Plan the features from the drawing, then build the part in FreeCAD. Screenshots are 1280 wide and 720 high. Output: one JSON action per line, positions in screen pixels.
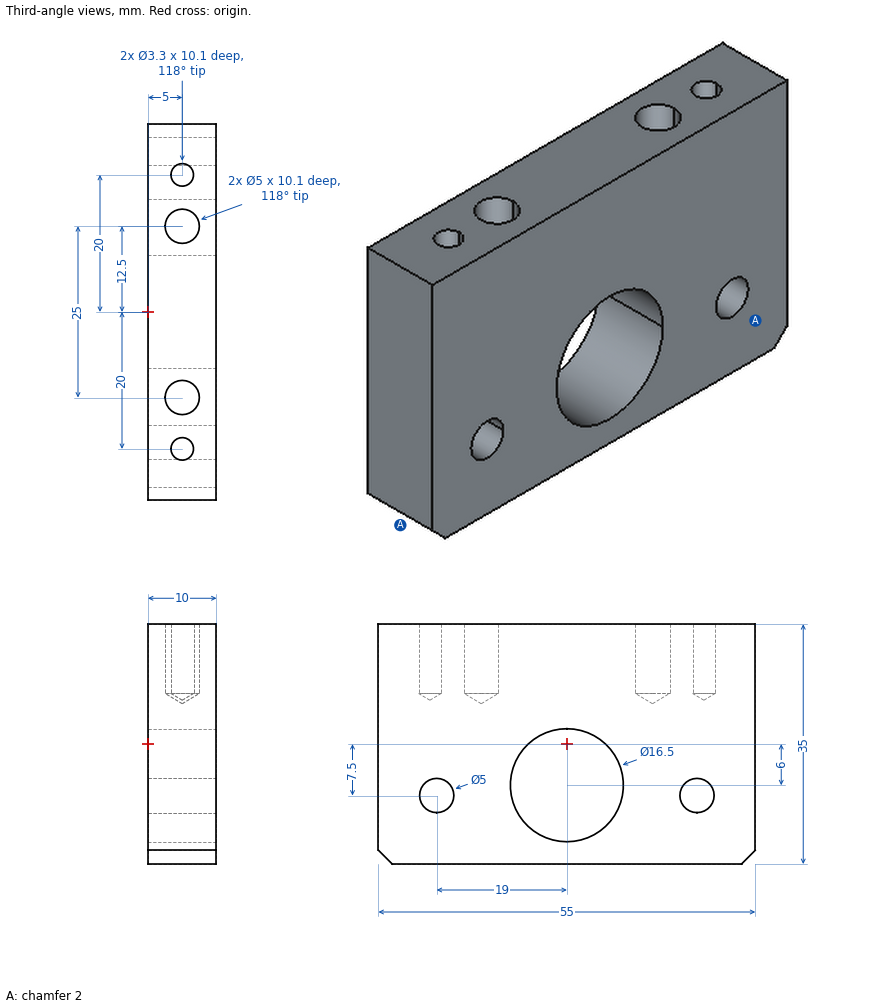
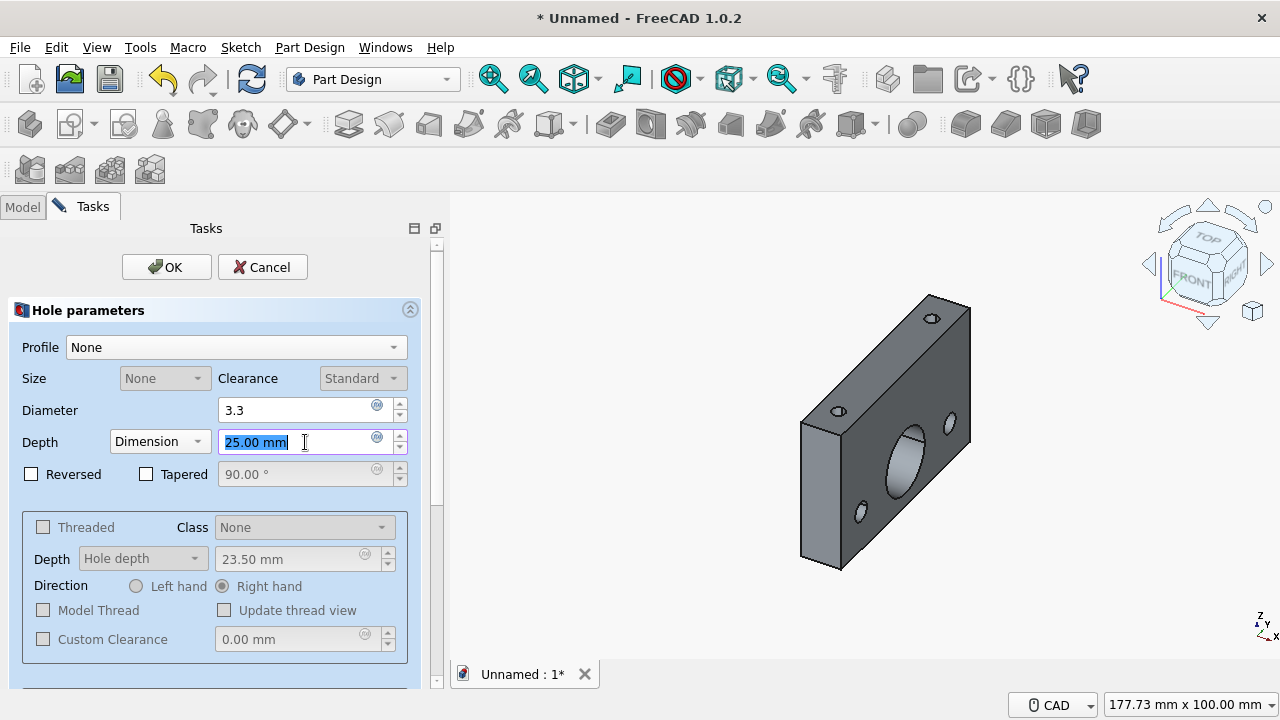
{"action": "type", "text": "10.1"}
{"action": "key", "text": "Tab"}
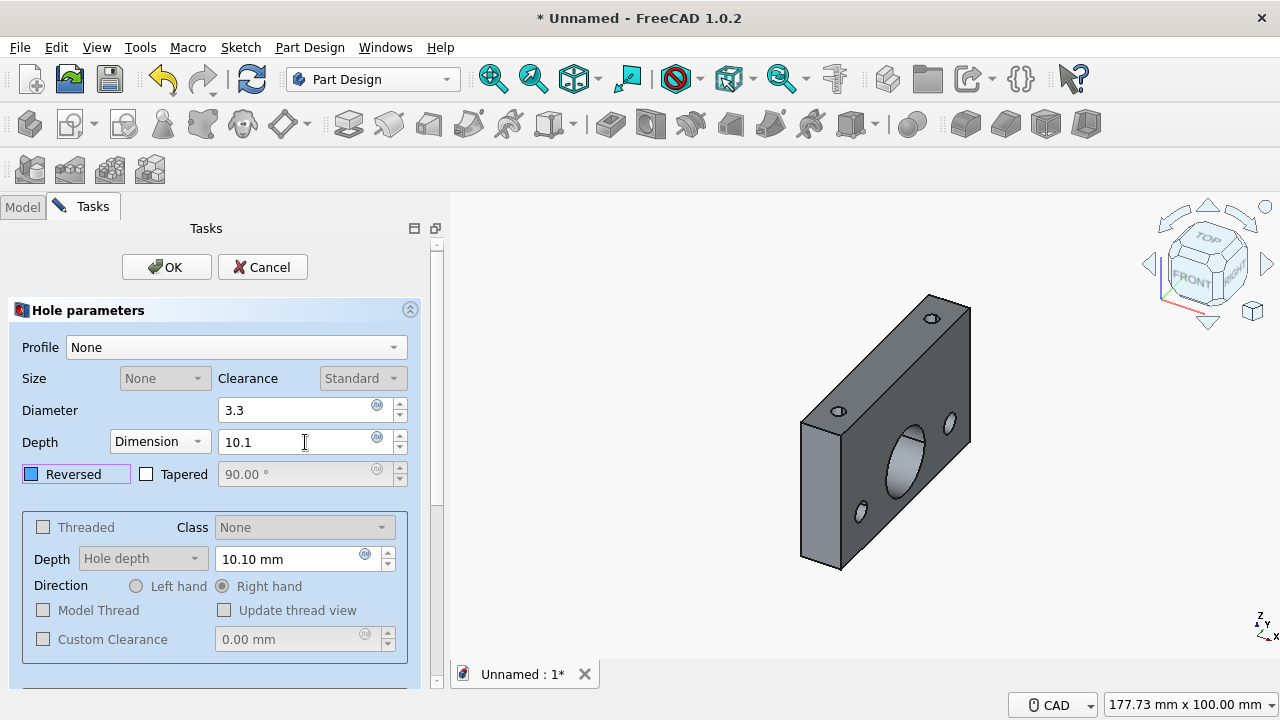
{"action": "left_click", "coordinate": [167, 267]}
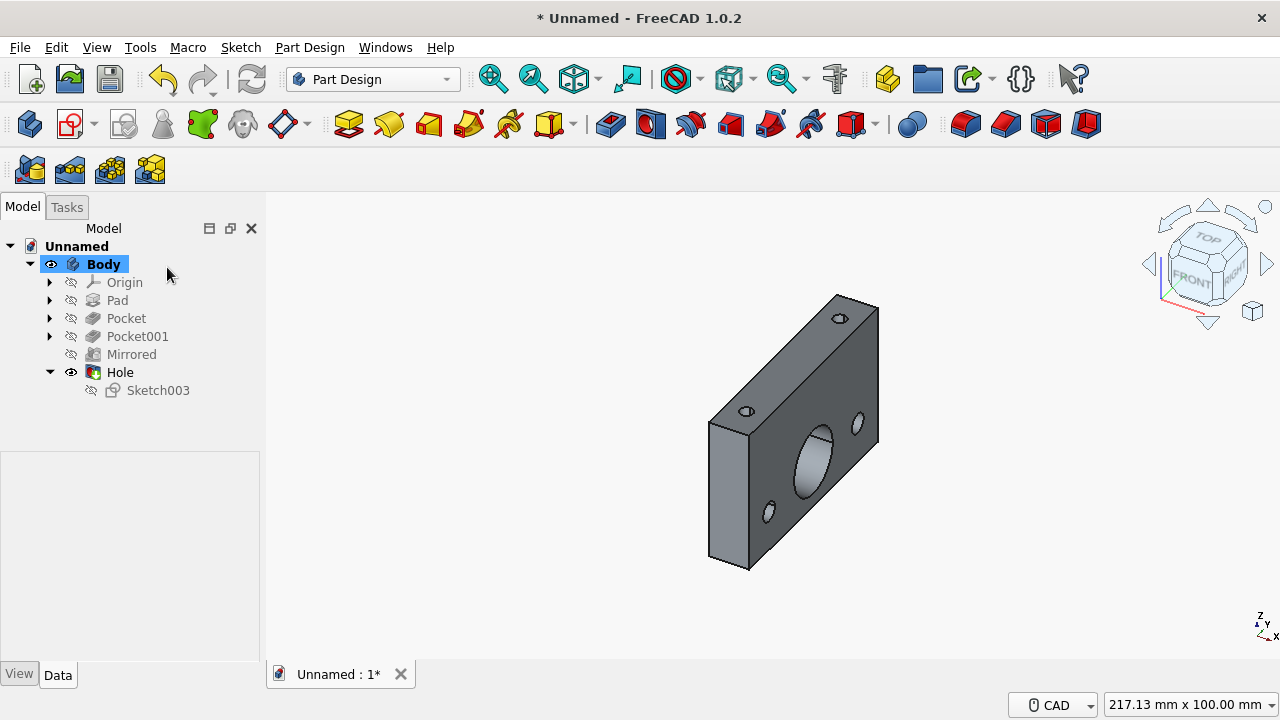
{"action": "left_click", "coordinate": [812, 346]}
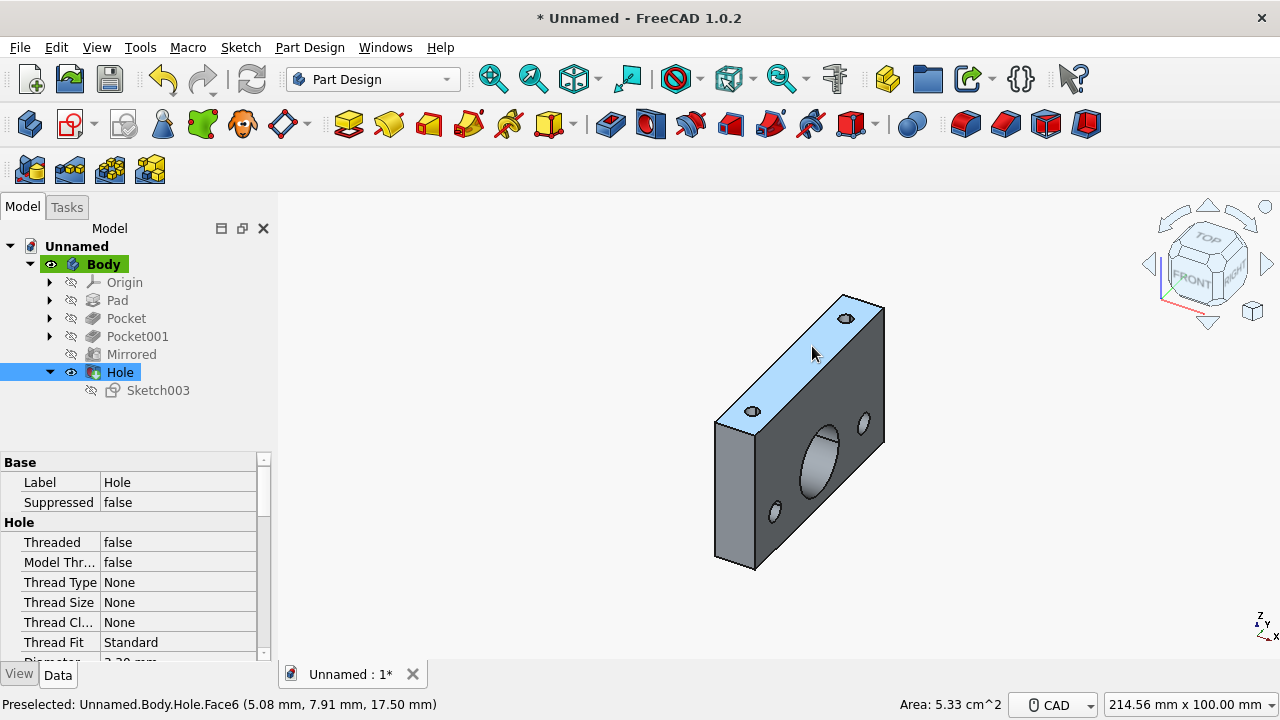
{"action": "left_click", "coordinate": [70, 124]}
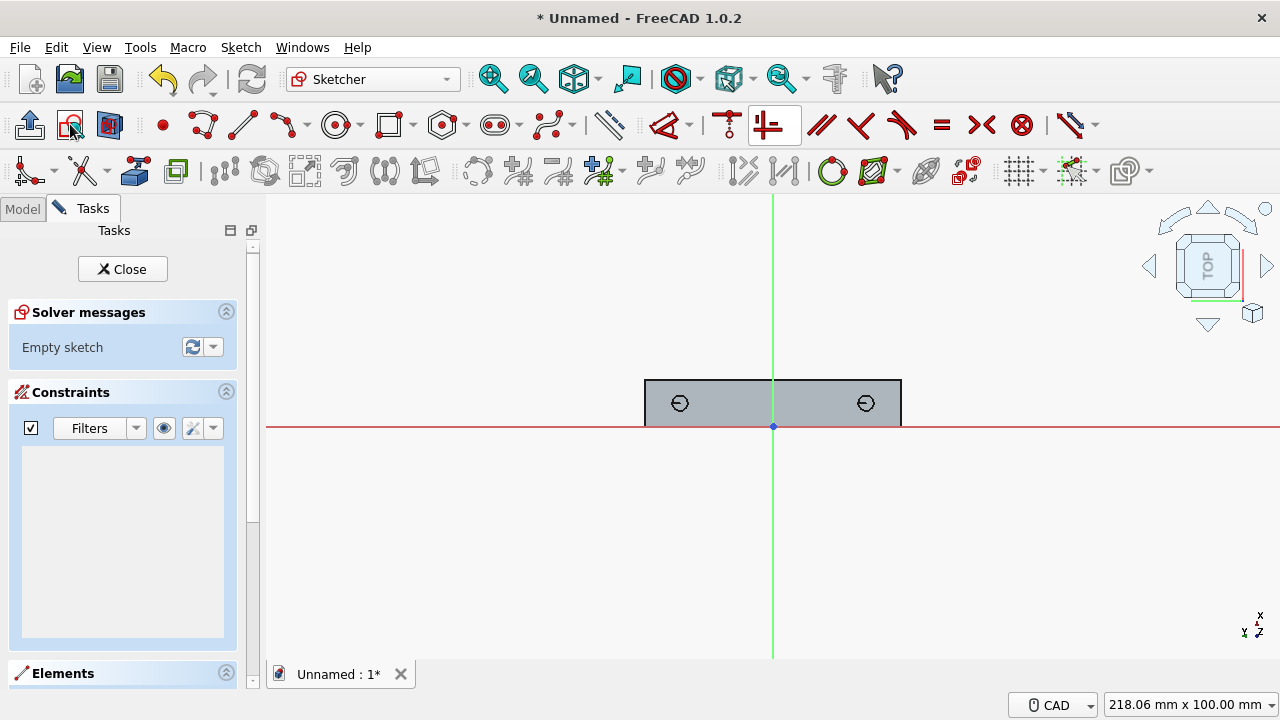
{"action": "scroll", "coordinate": [795, 403], "scroll_direction": "up", "scroll_amount": 7}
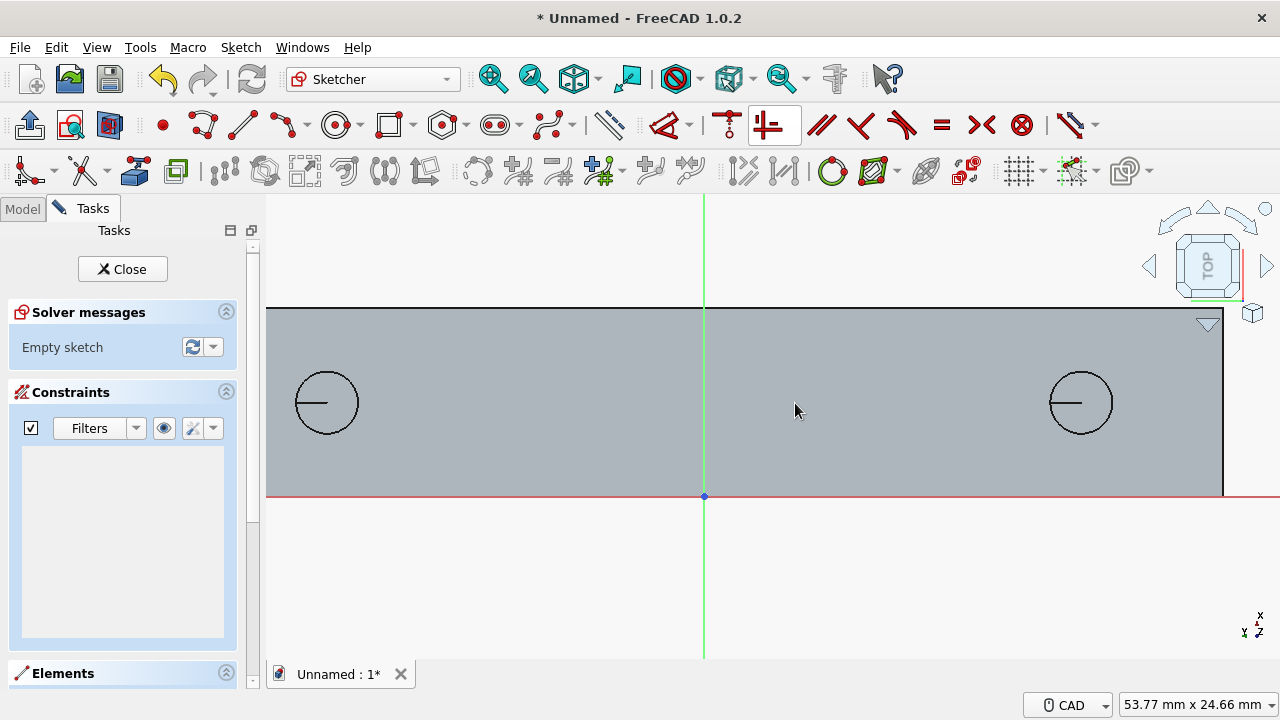
{"action": "key", "text": "g c"}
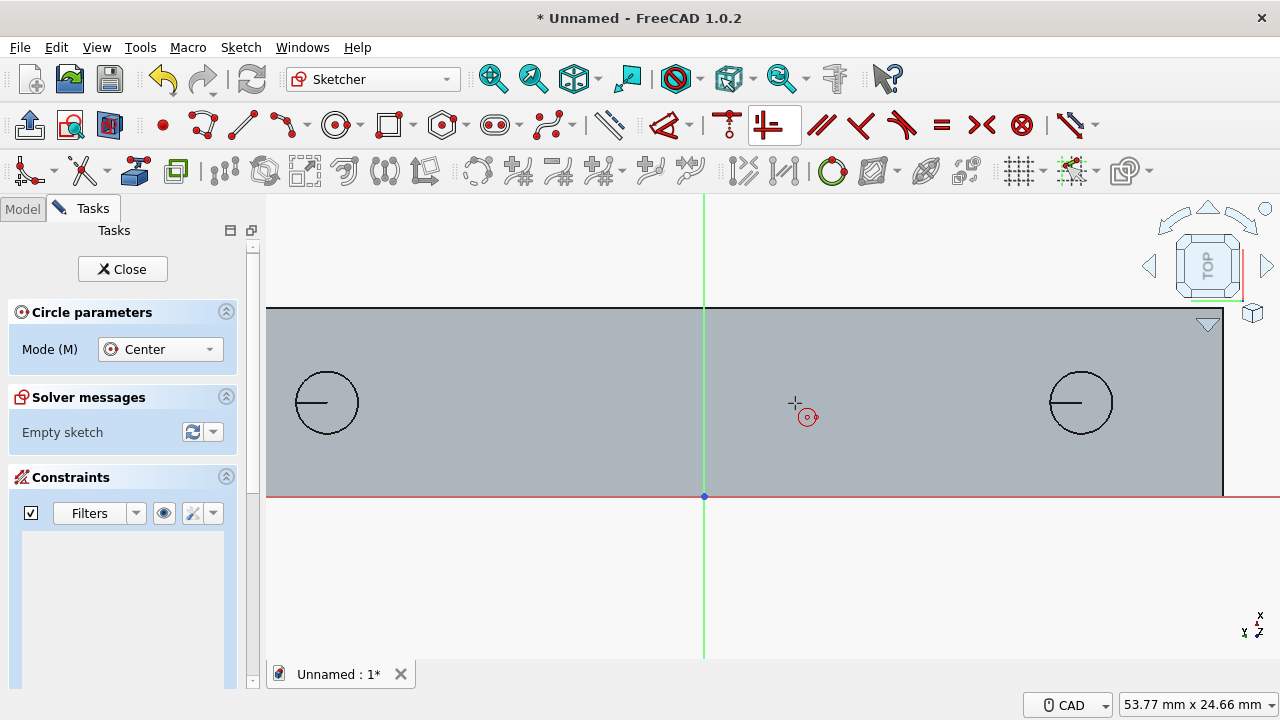
{"action": "left_click", "coordinate": [468, 403]}
{"action": "mouse_move", "coordinate": [502, 369]}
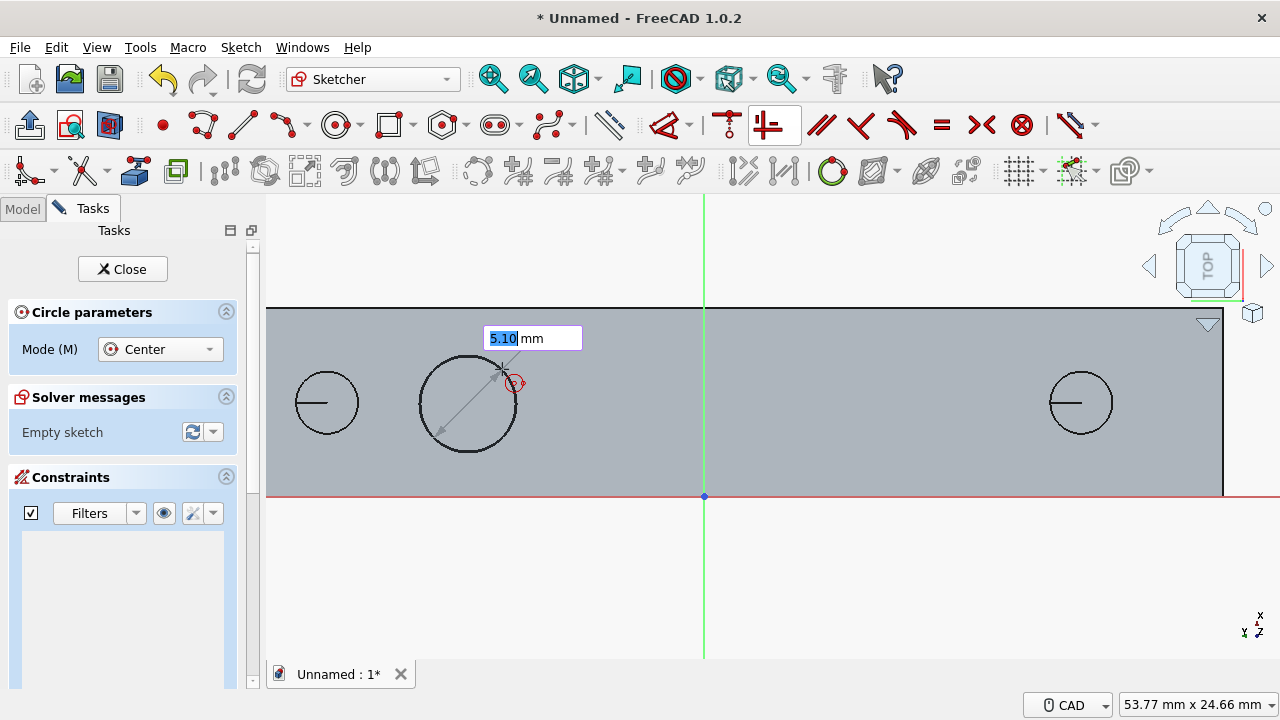
{"action": "type", "text": "5"}
{"action": "key", "text": "Return"}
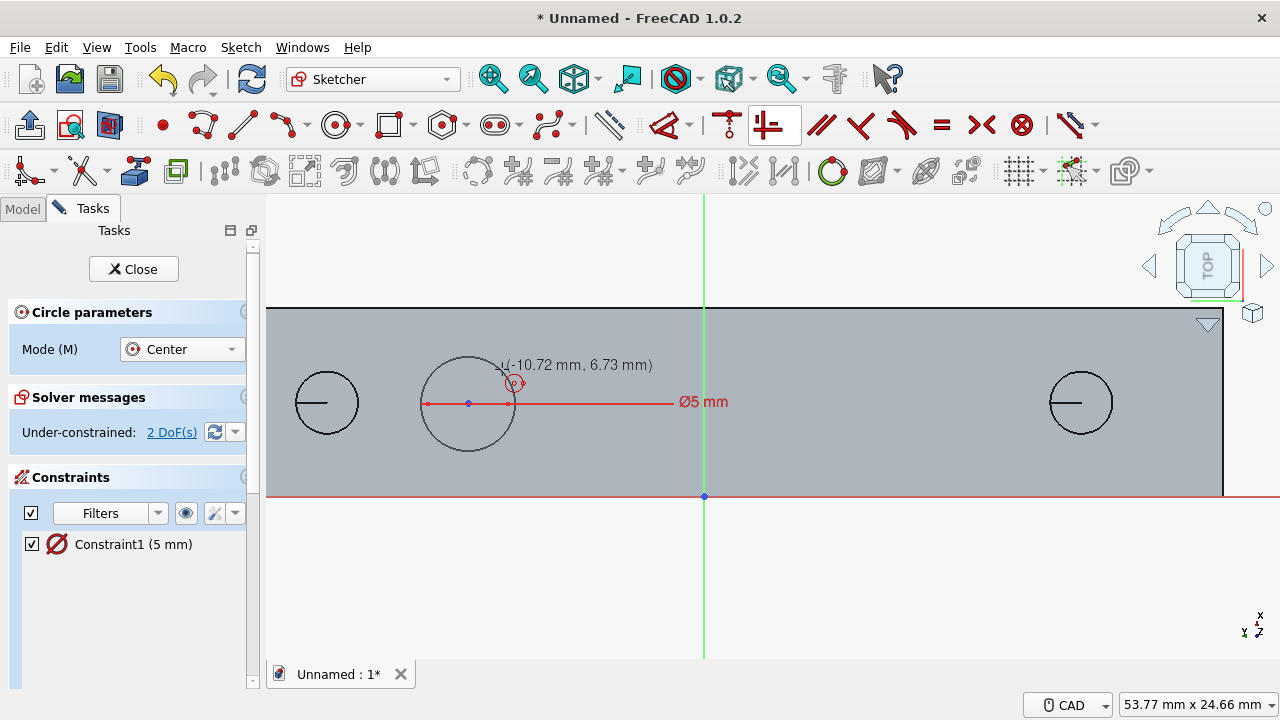
{"action": "left_click", "coordinate": [940, 403]}
{"action": "mouse_move", "coordinate": [973, 369]}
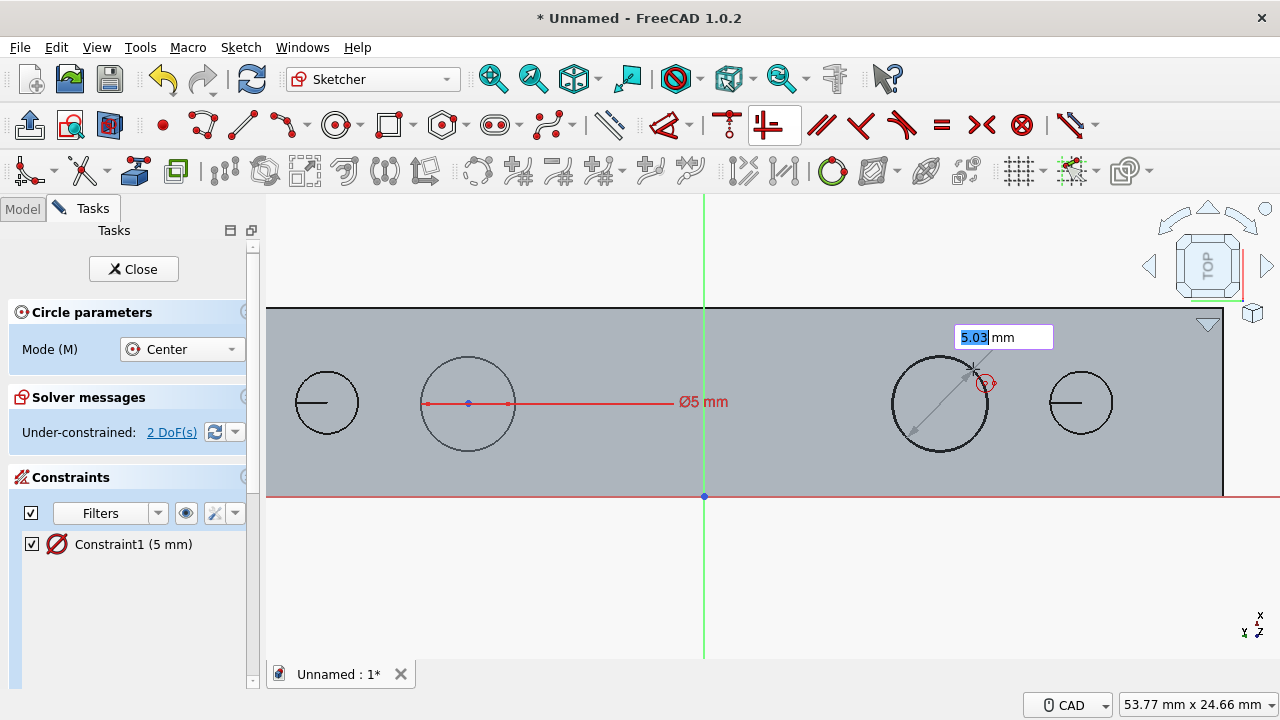
{"action": "type", "text": "5"}
{"action": "key", "text": "Return"}
{"action": "key", "text": "Escape"}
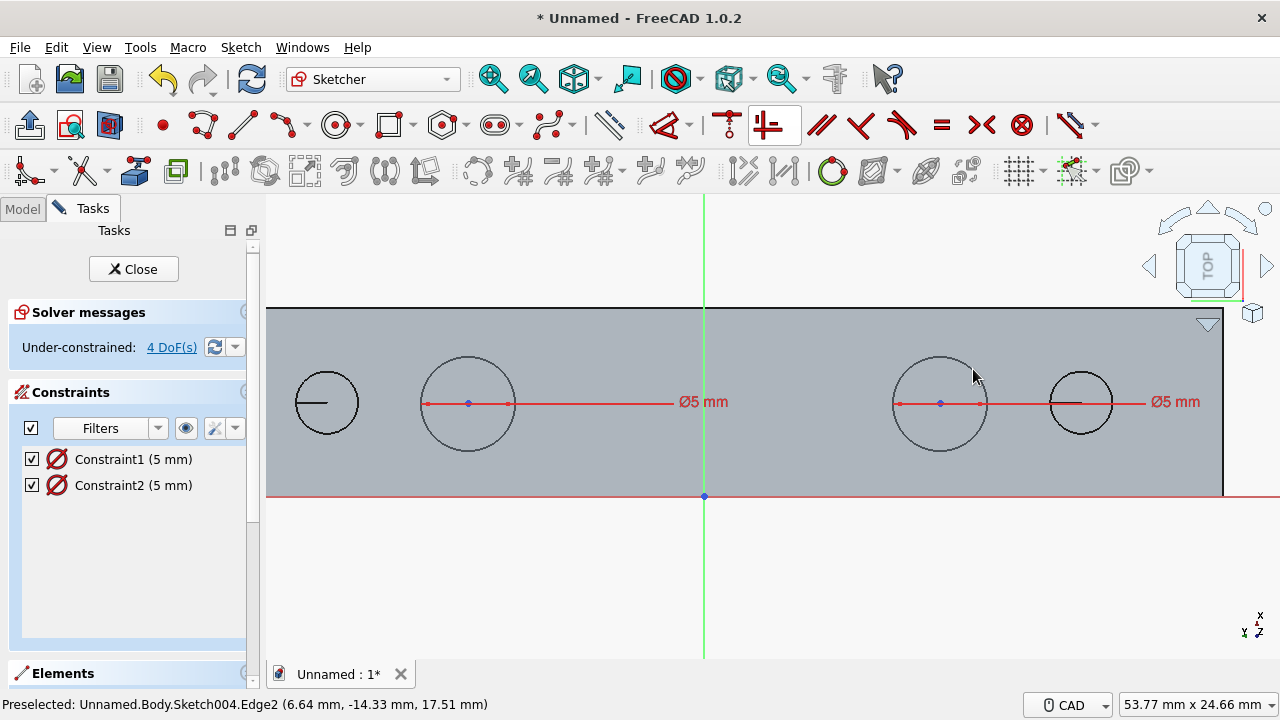
{"action": "left_click", "coordinate": [468, 404]}